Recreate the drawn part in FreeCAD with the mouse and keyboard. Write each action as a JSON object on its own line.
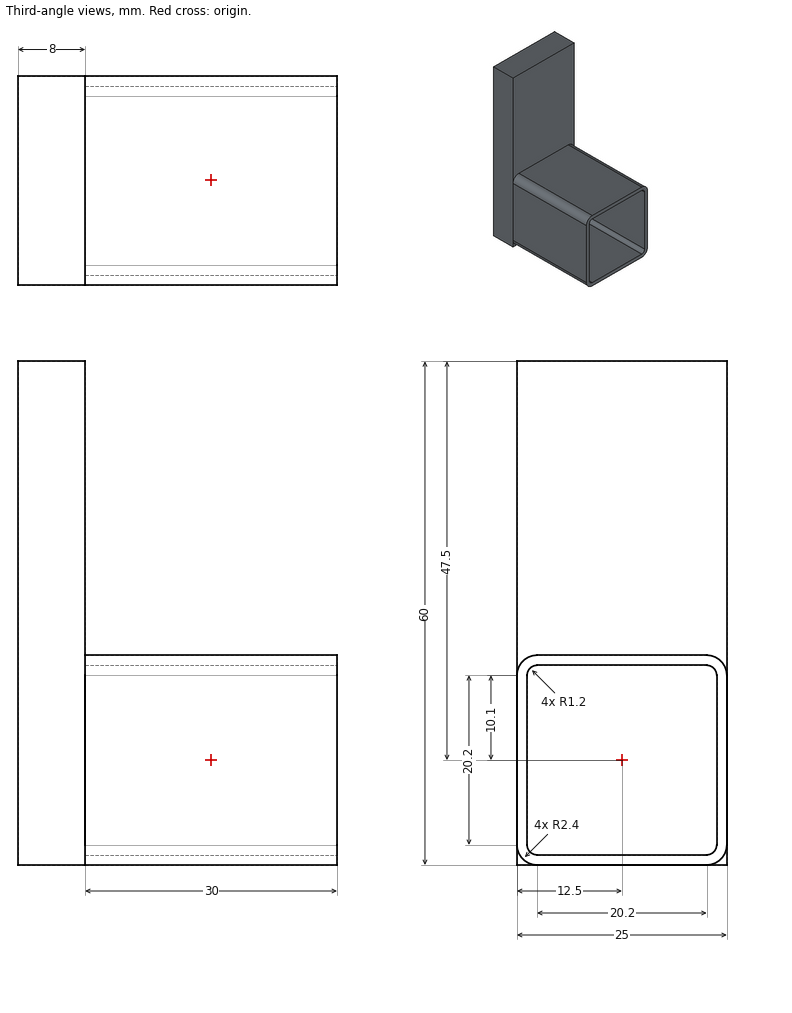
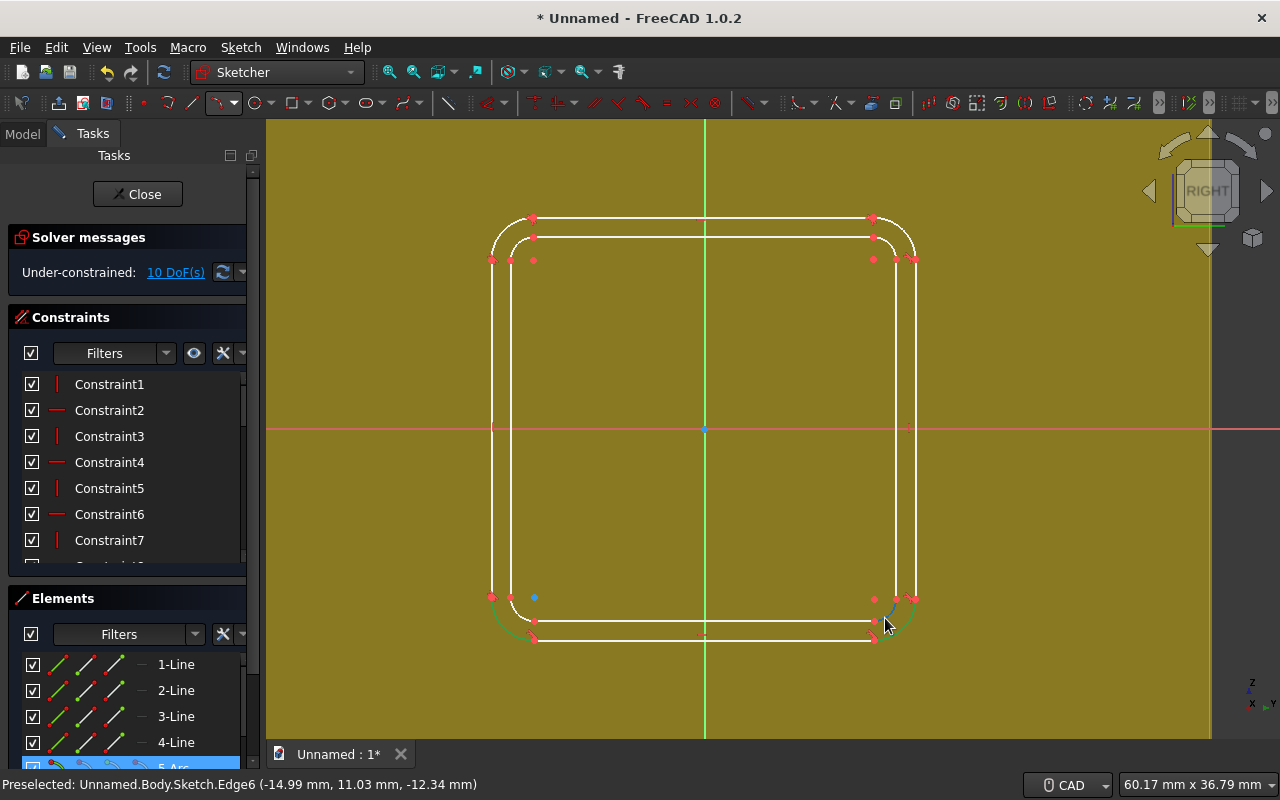
{"action": "left_click", "coordinate": [911, 241]}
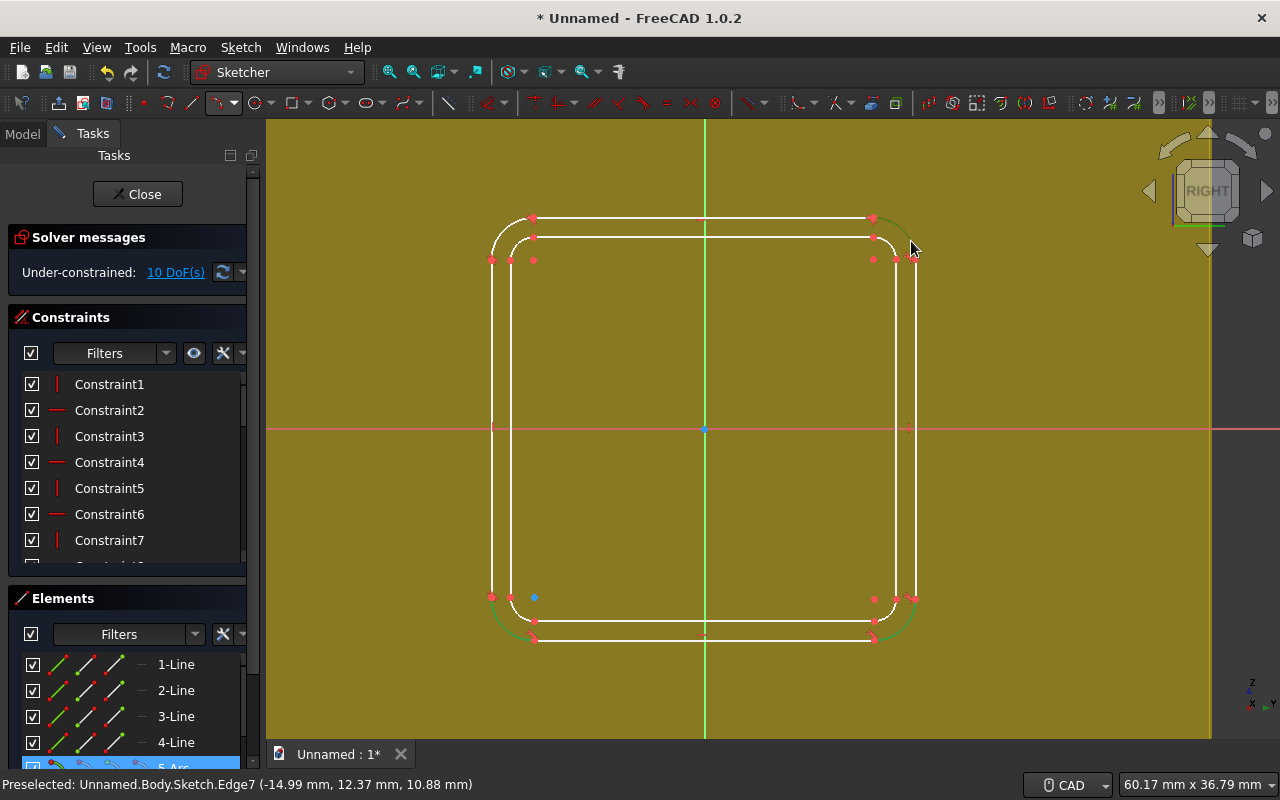
{"action": "left_click", "coordinate": [515, 222]}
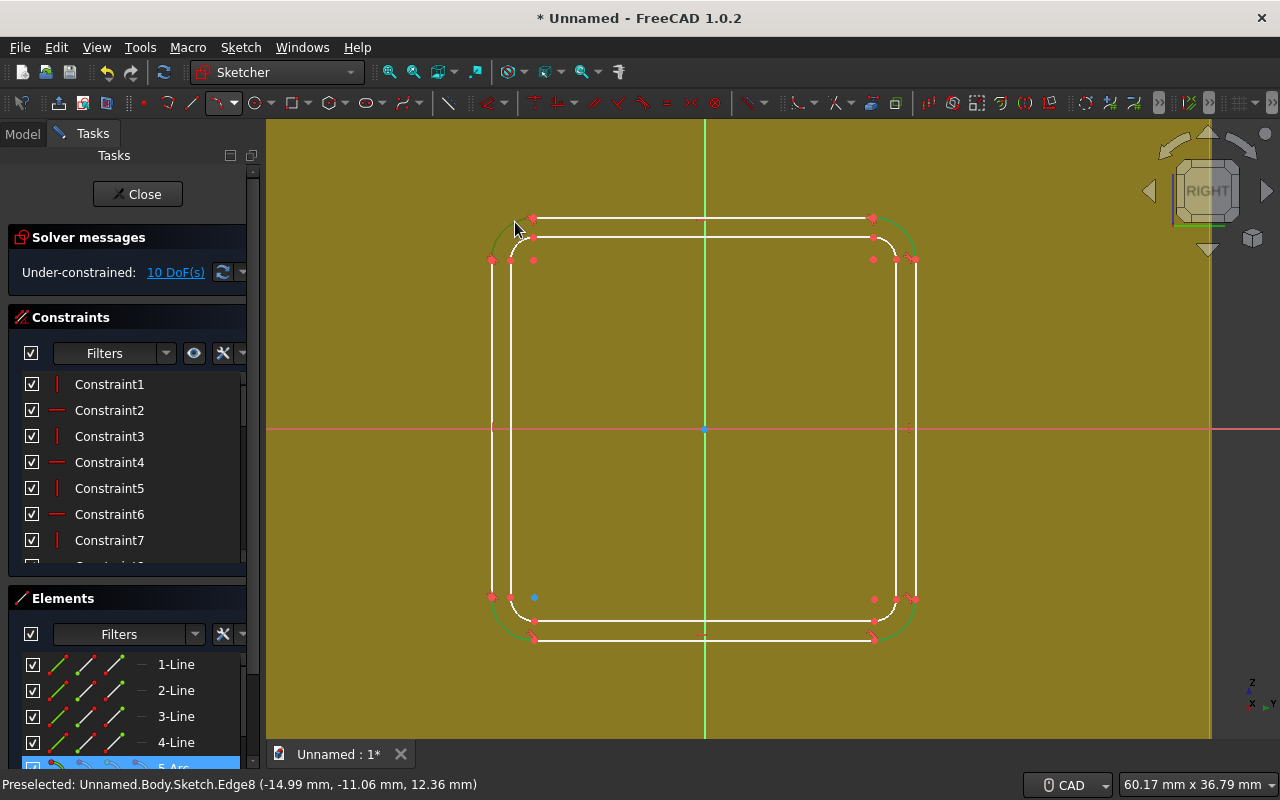
{"action": "left_click", "coordinate": [668, 104]}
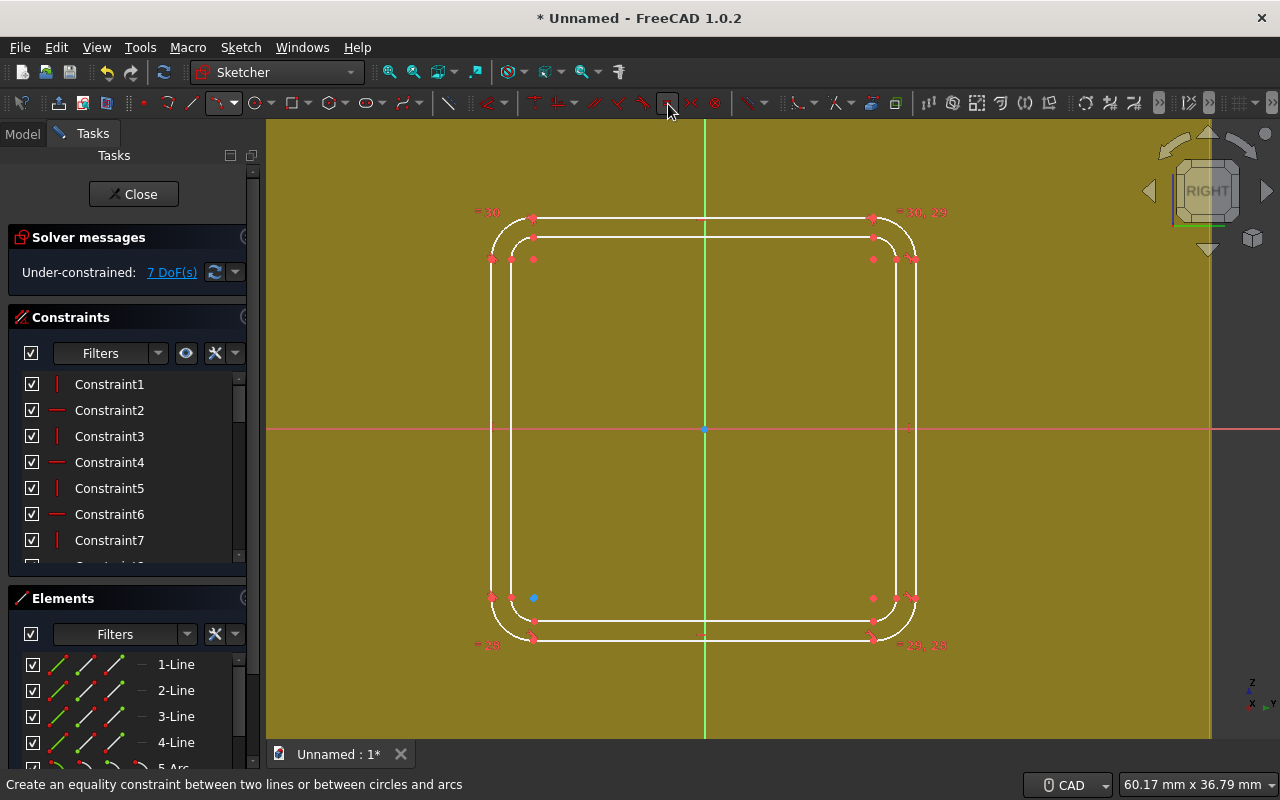
{"action": "scroll", "coordinate": [523, 240], "scroll_direction": "up", "scroll_amount": 2}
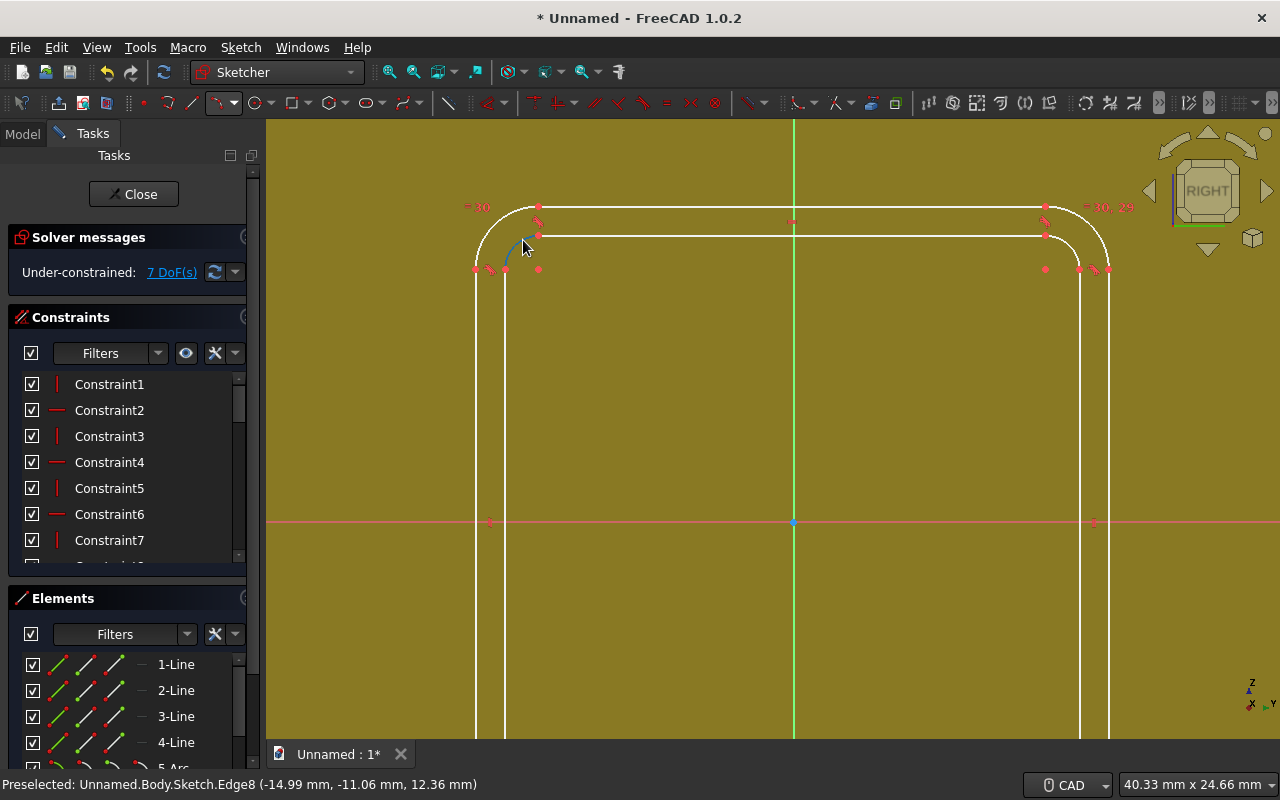
{"action": "left_click", "coordinate": [524, 240]}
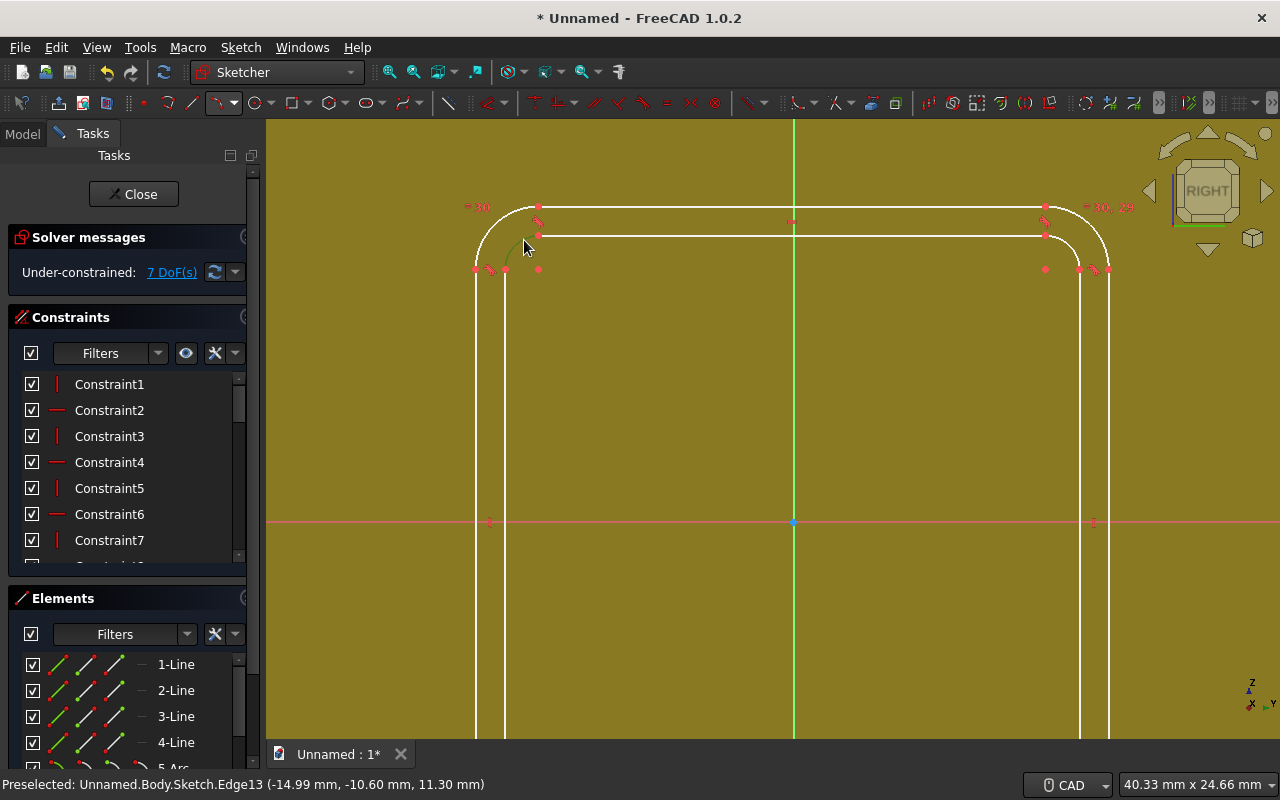
{"action": "scroll", "coordinate": [523, 240], "scroll_direction": "down", "scroll_amount": 2}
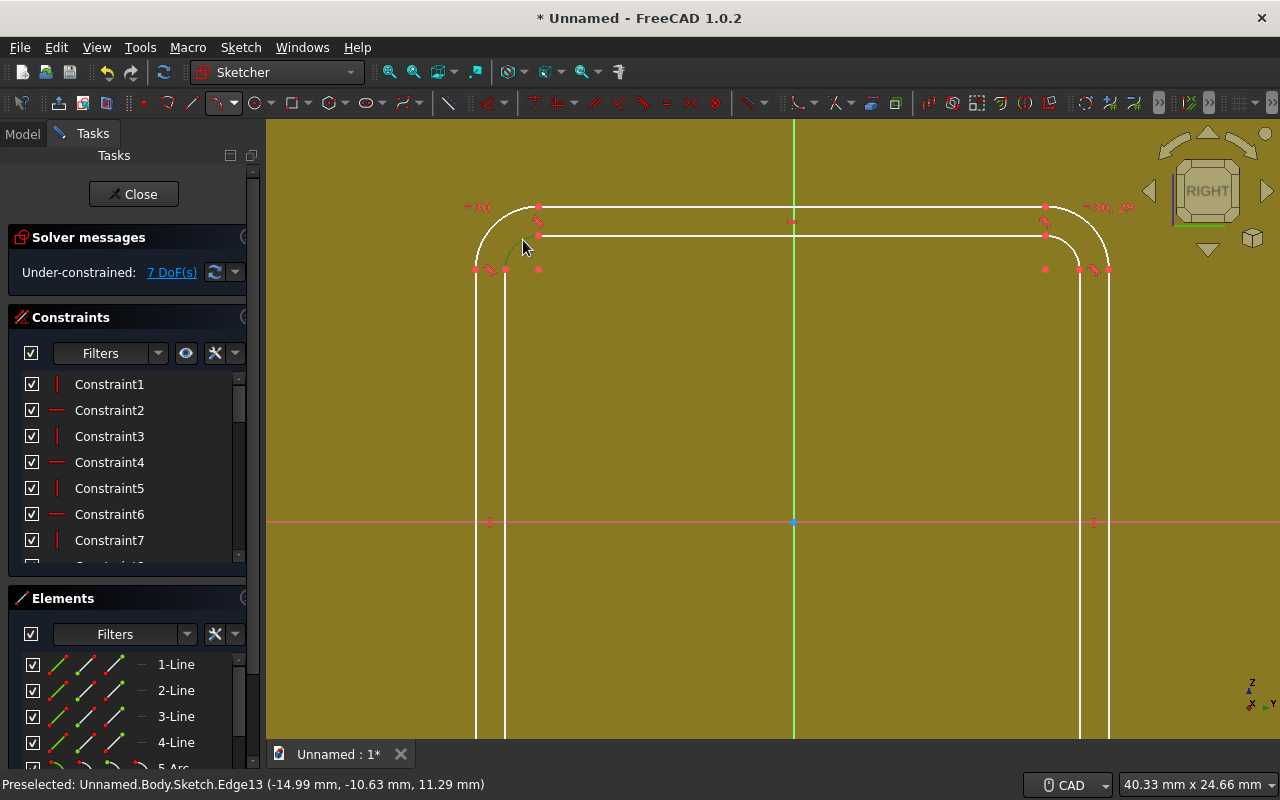
{"action": "scroll", "coordinate": [514, 608], "scroll_direction": "up", "scroll_amount": 2}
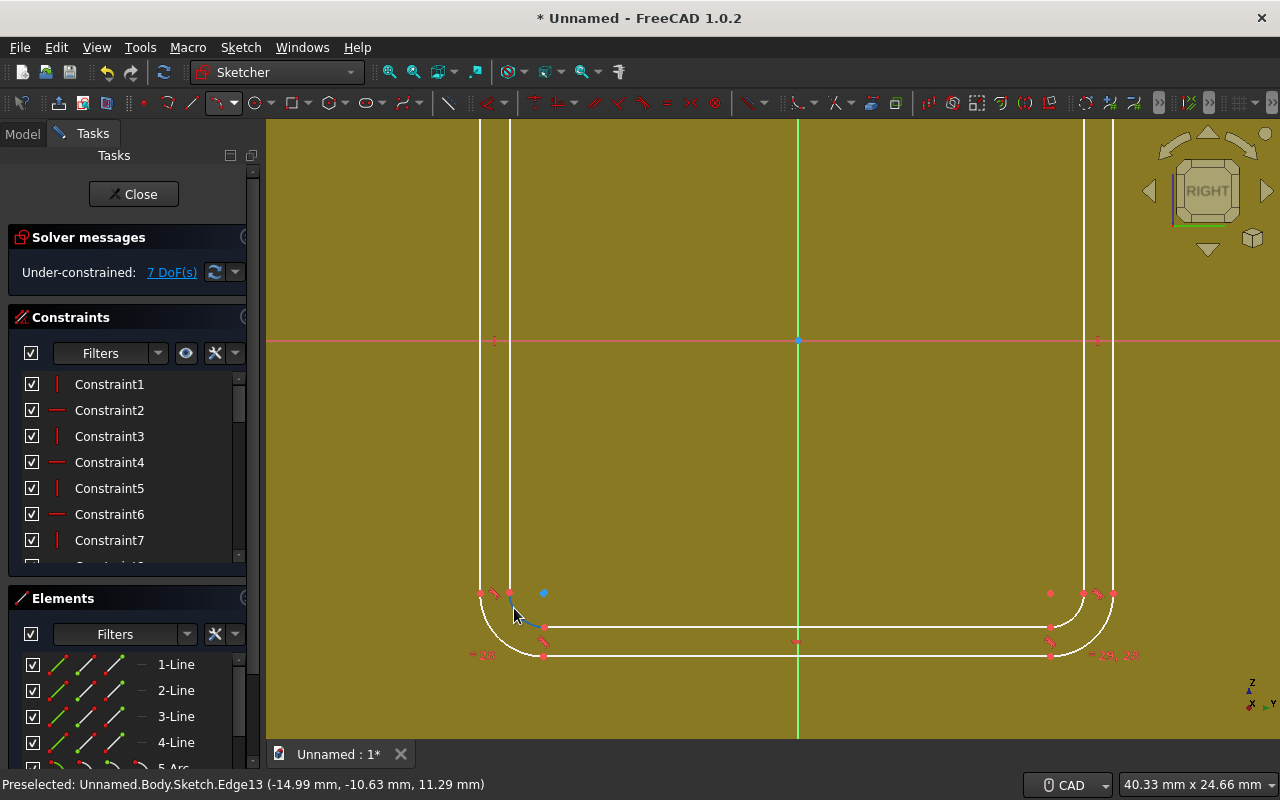
{"action": "left_click", "coordinate": [513, 608]}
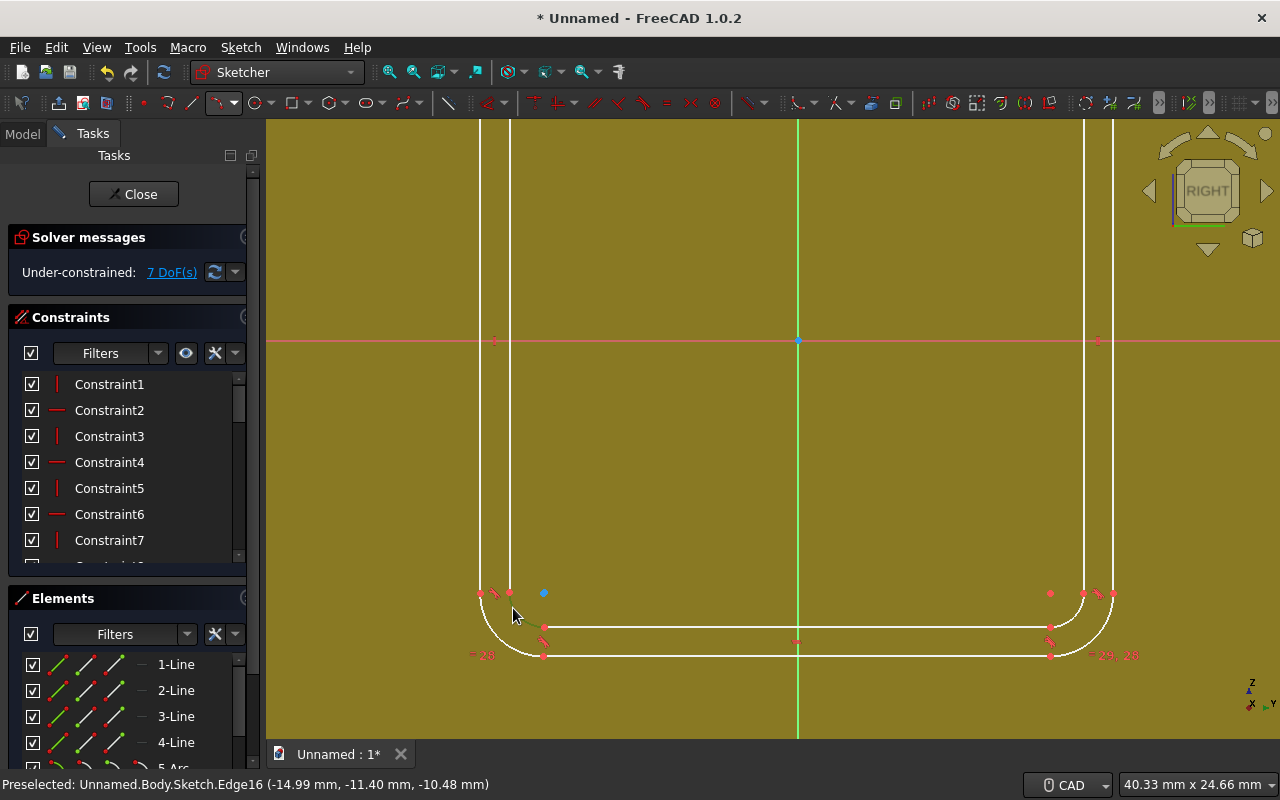
{"action": "key", "text": "e"}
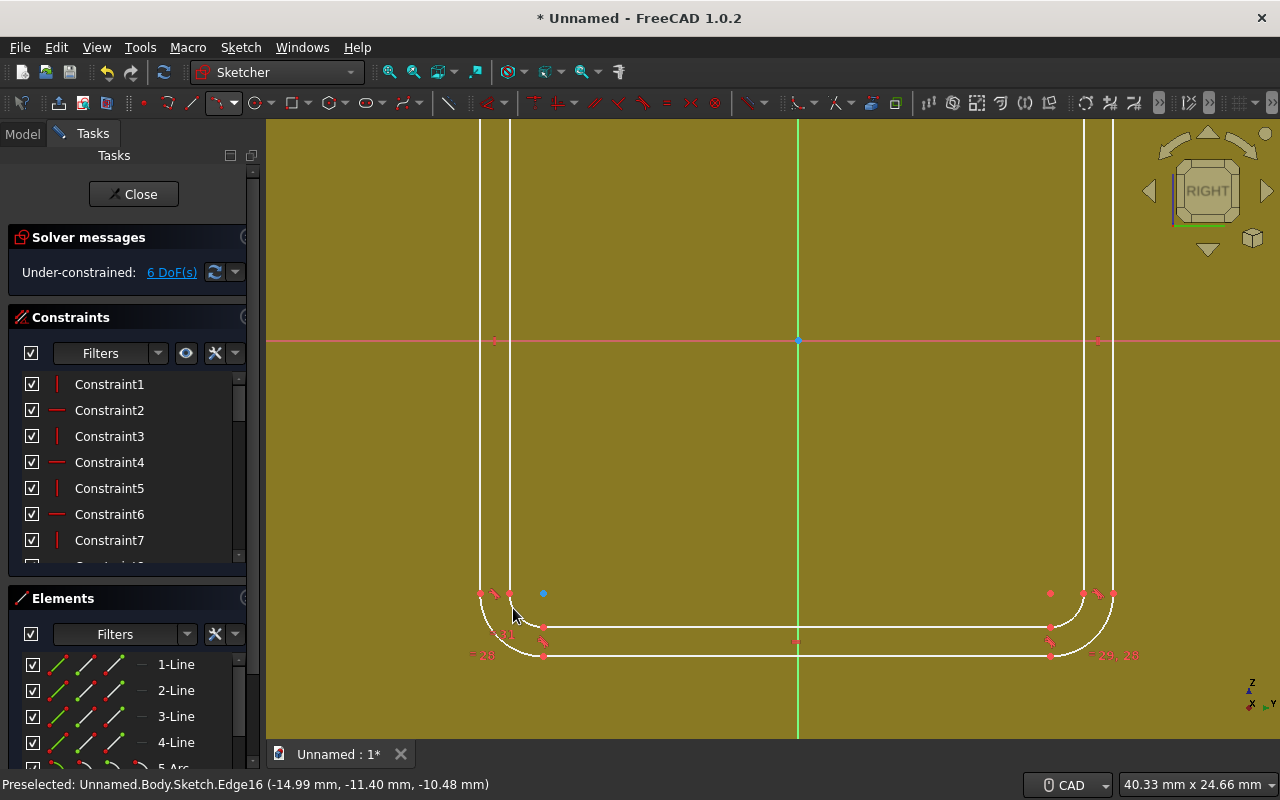
{"action": "left_click", "coordinate": [488, 104]}